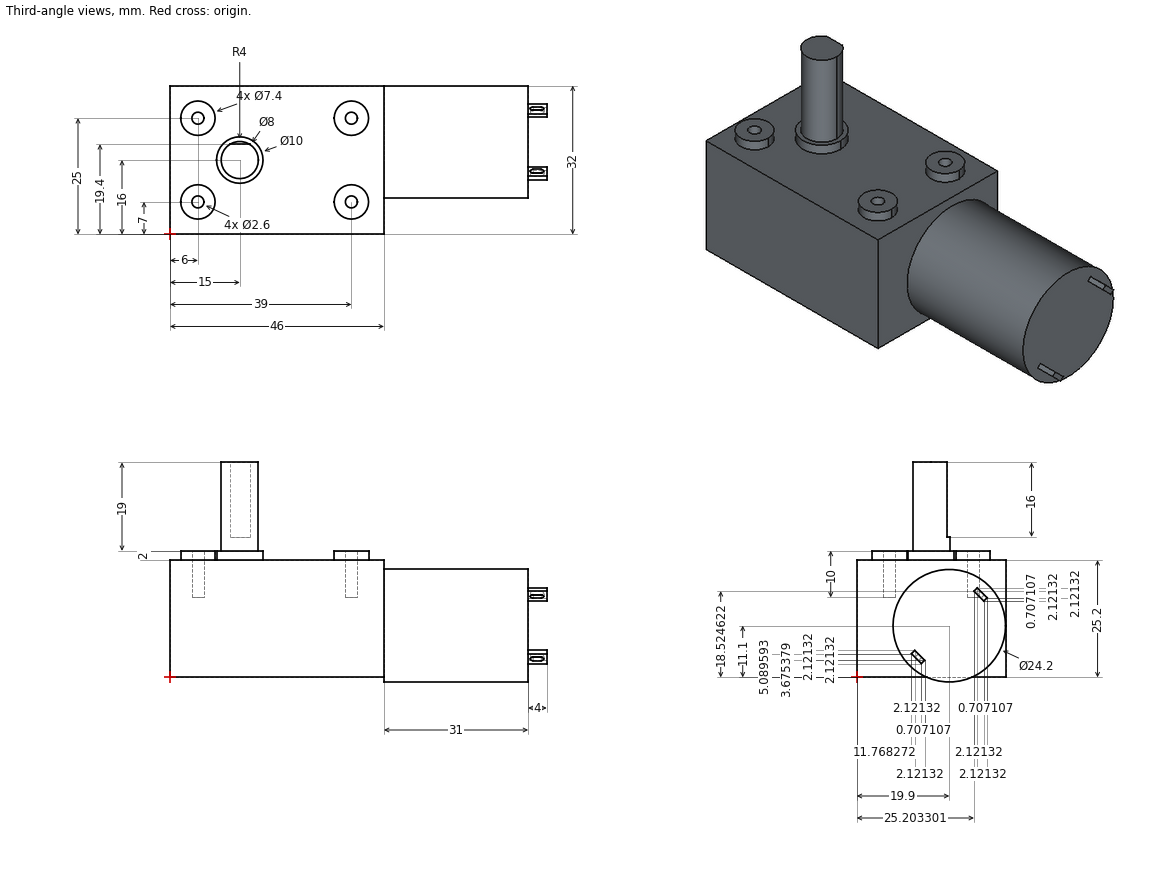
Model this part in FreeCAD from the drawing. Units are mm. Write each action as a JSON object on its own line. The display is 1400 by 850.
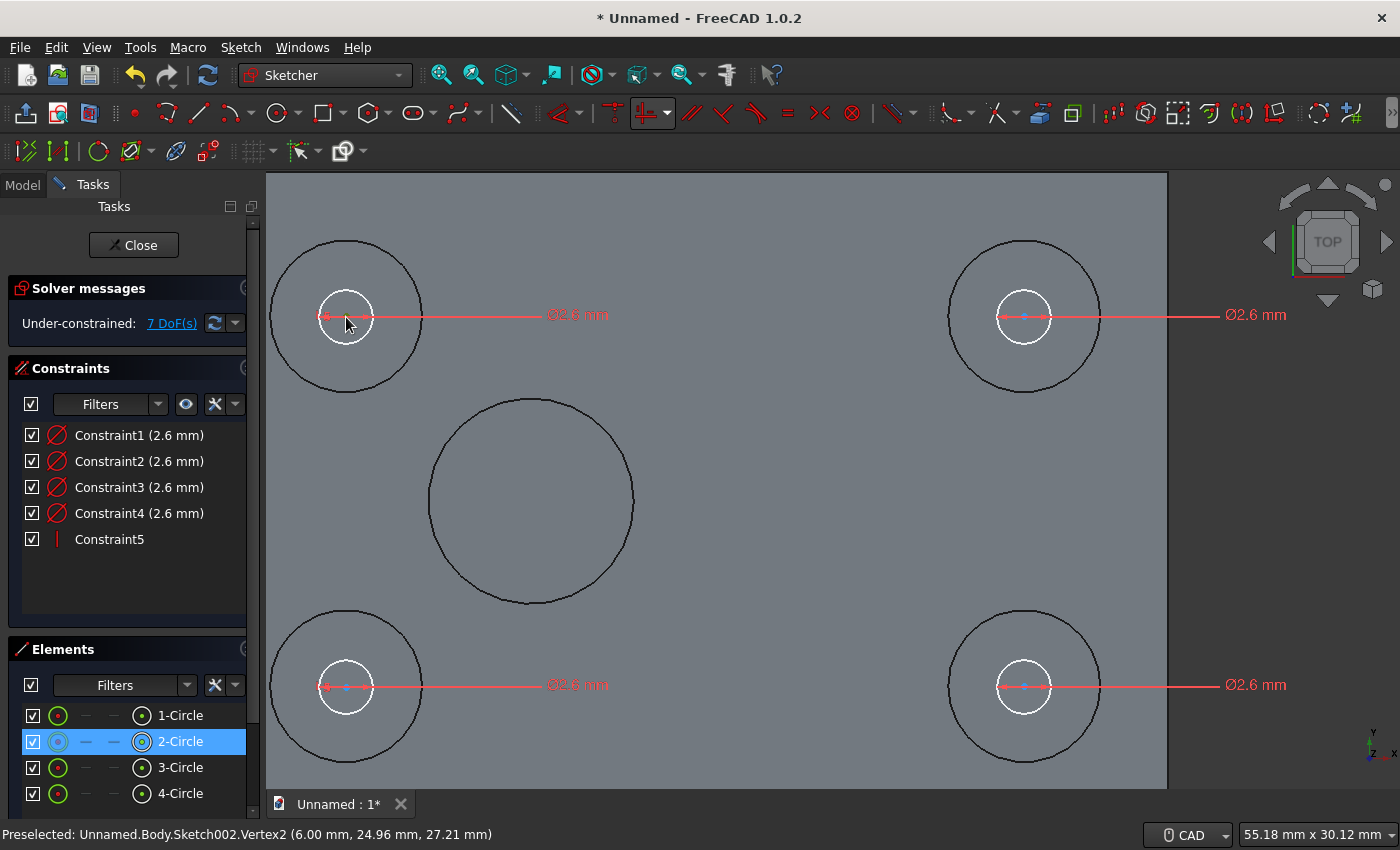
{"action": "left_click", "coordinate": [1024, 317]}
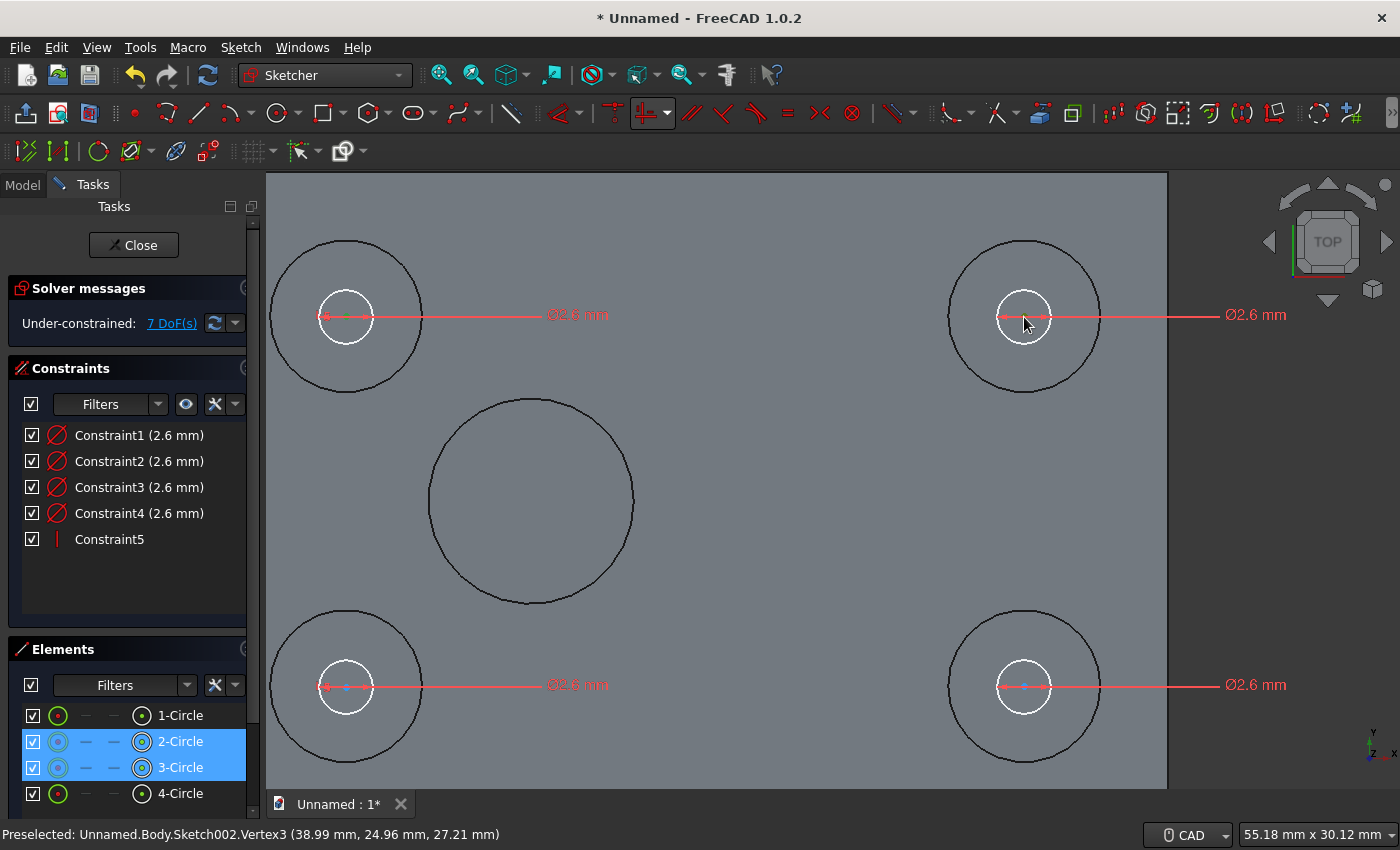
{"action": "key", "text": "h"}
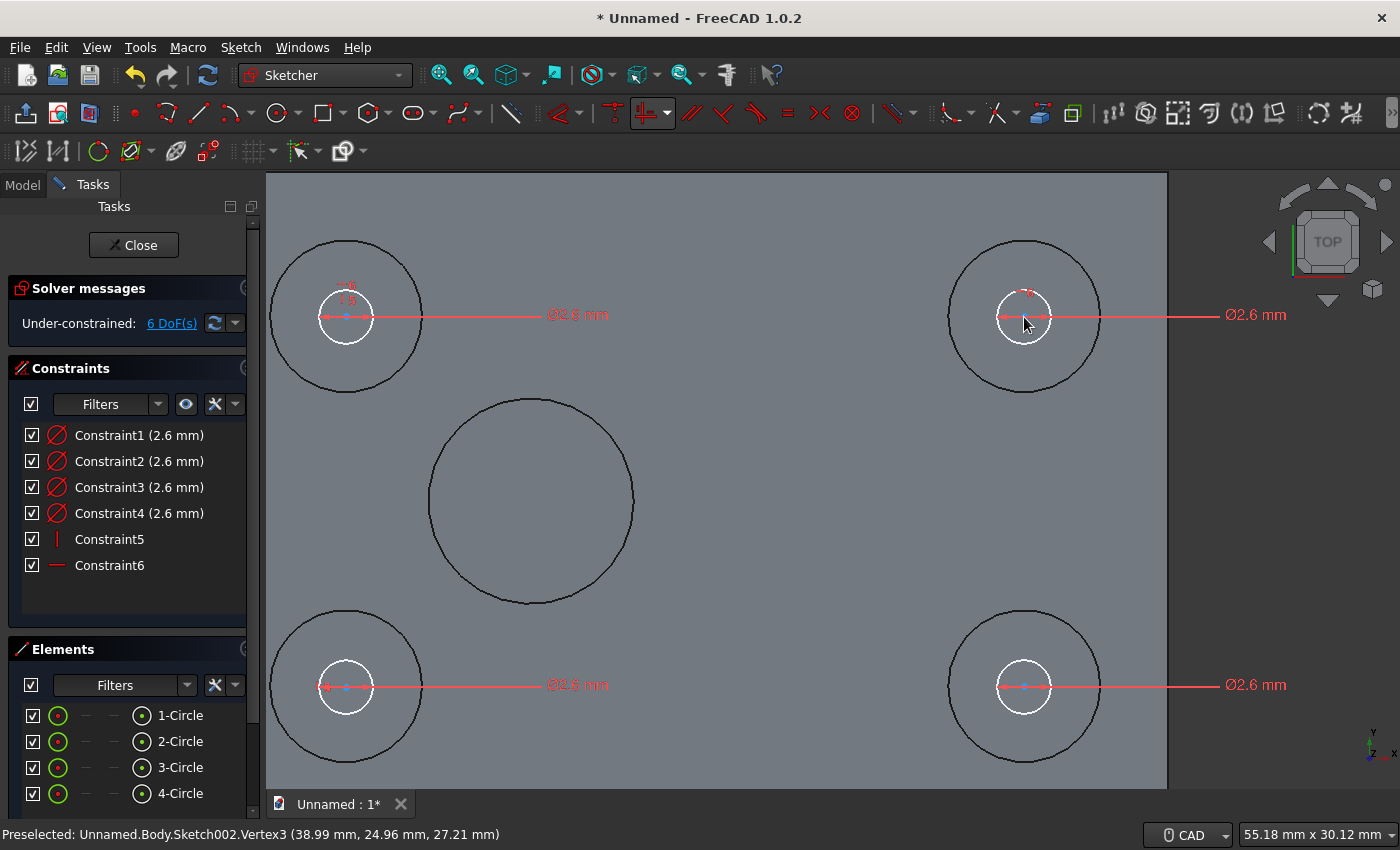
{"action": "left_click", "coordinate": [1024, 317]}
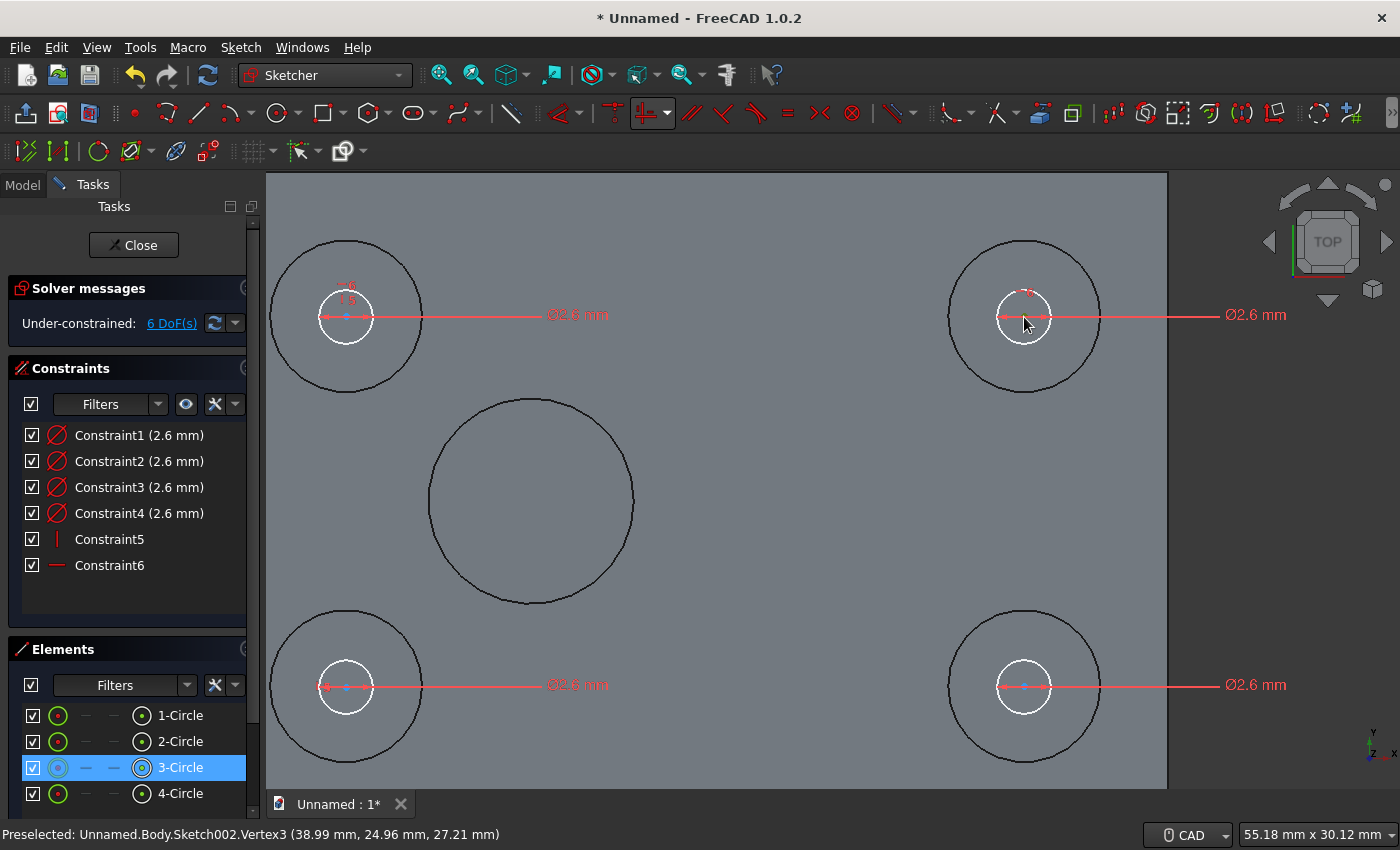
{"action": "left_click", "coordinate": [1024, 687]}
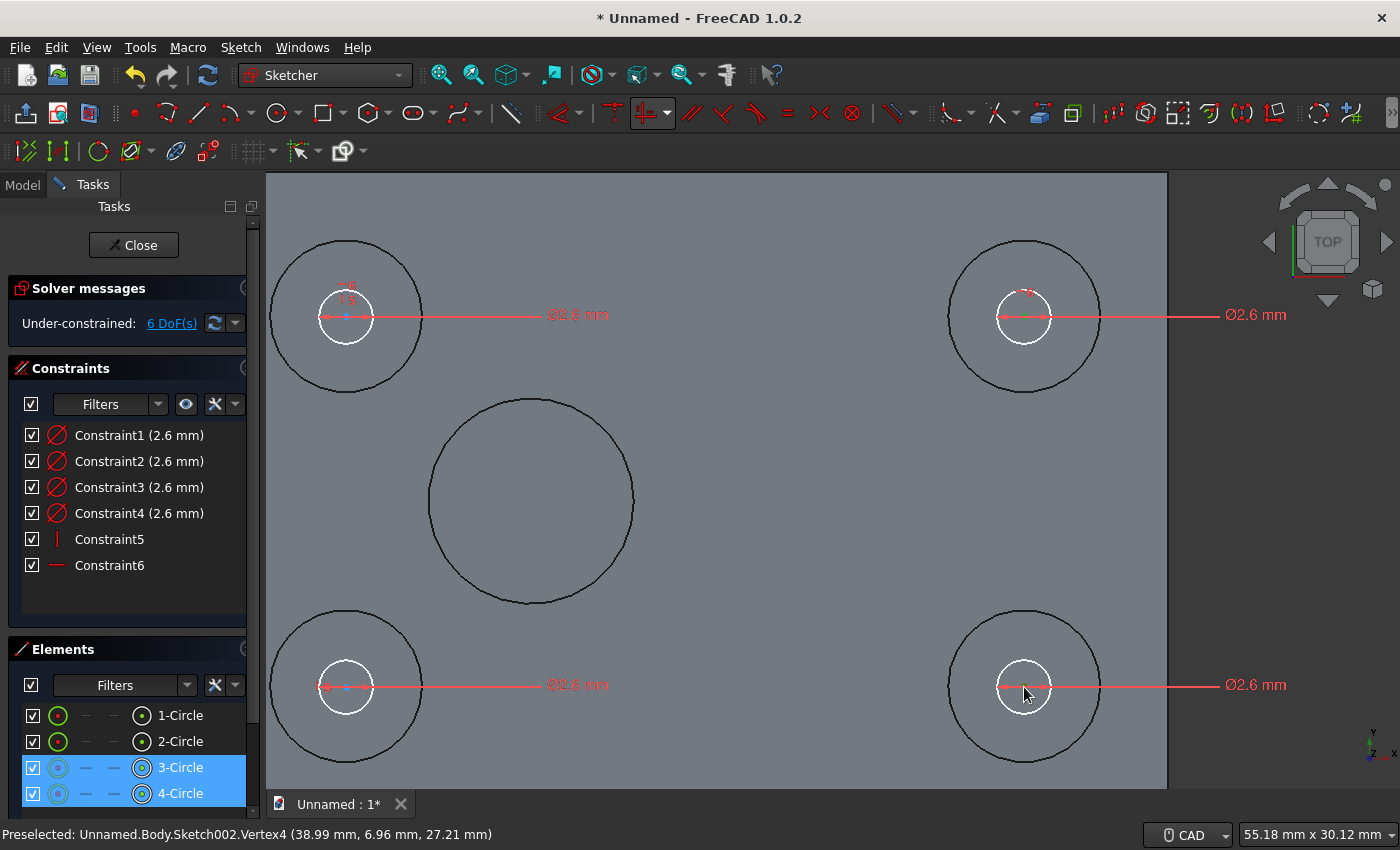
{"action": "key", "text": "v"}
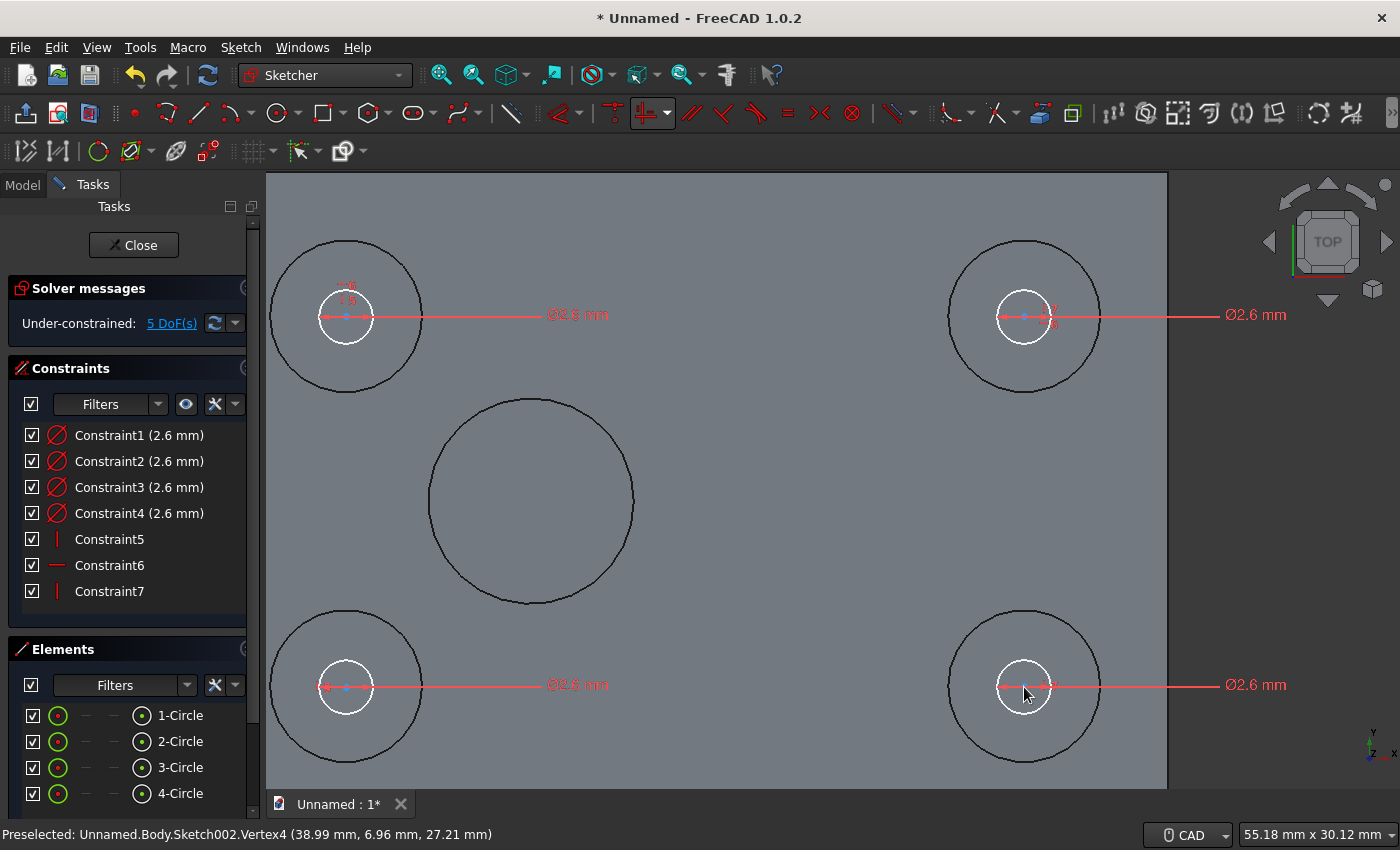
{"action": "left_click", "coordinate": [346, 687]}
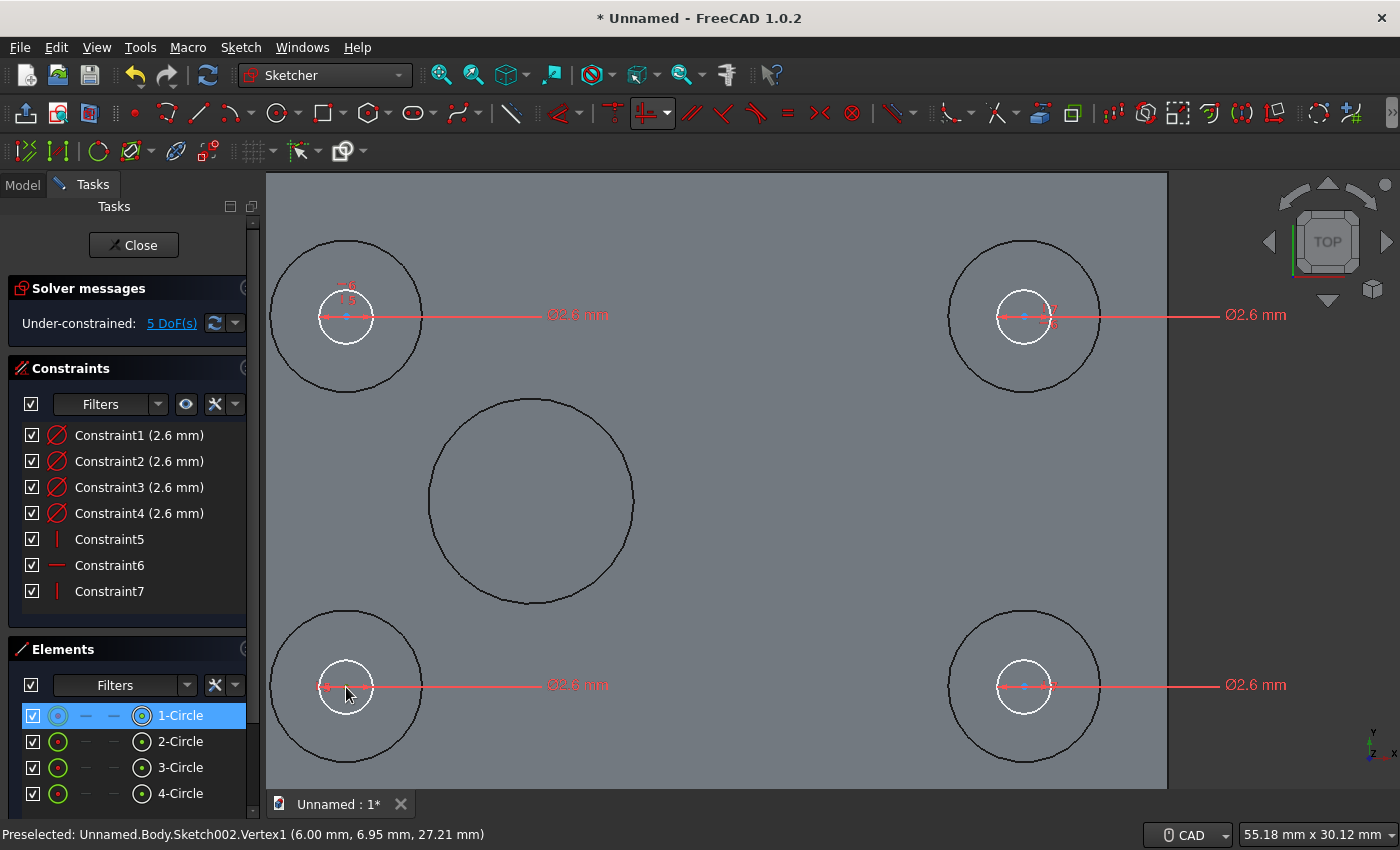
{"action": "left_click", "coordinate": [1024, 687]}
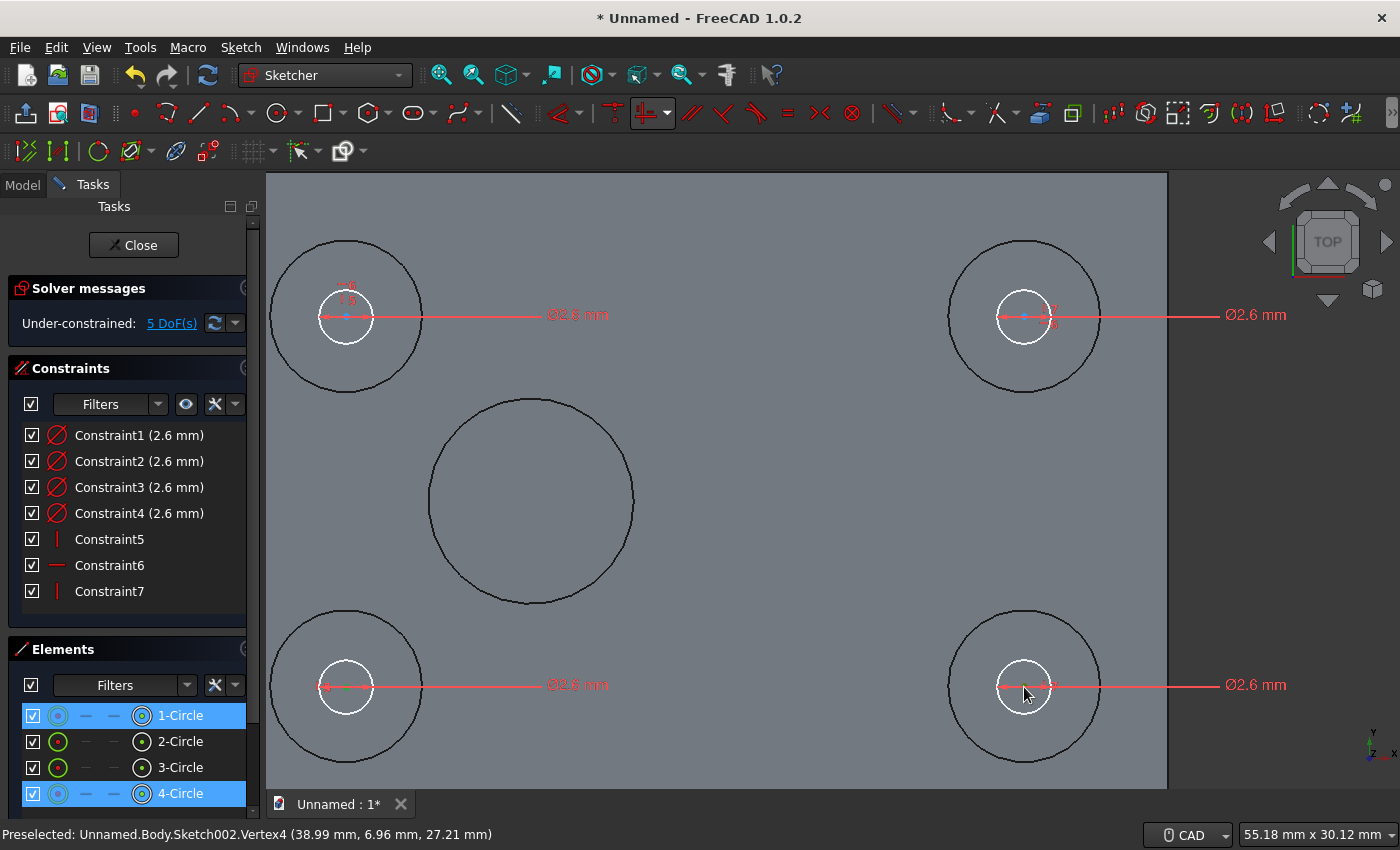
{"action": "key", "text": "h"}